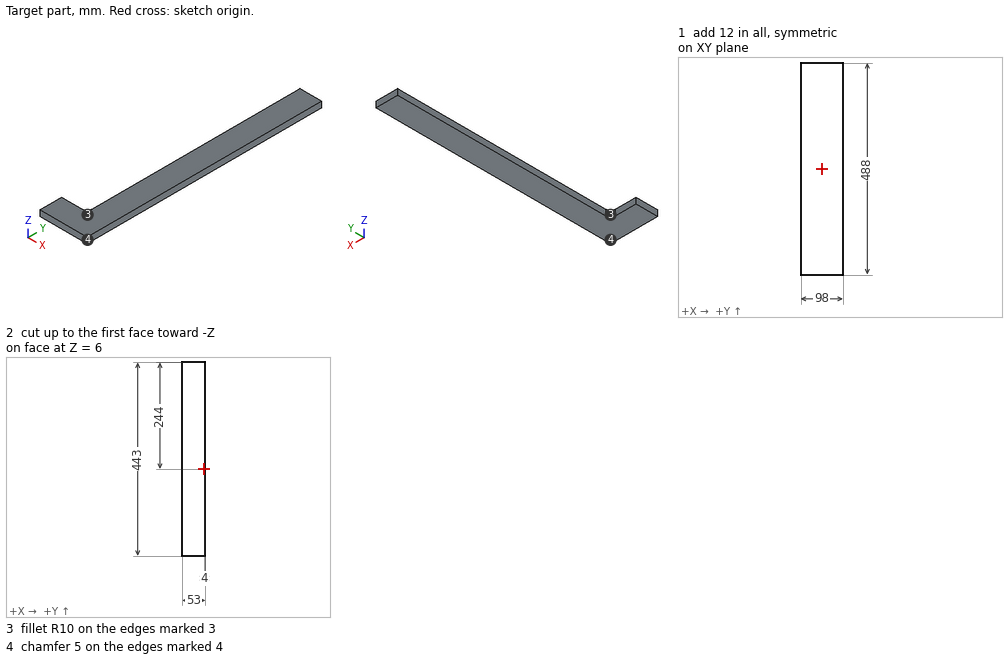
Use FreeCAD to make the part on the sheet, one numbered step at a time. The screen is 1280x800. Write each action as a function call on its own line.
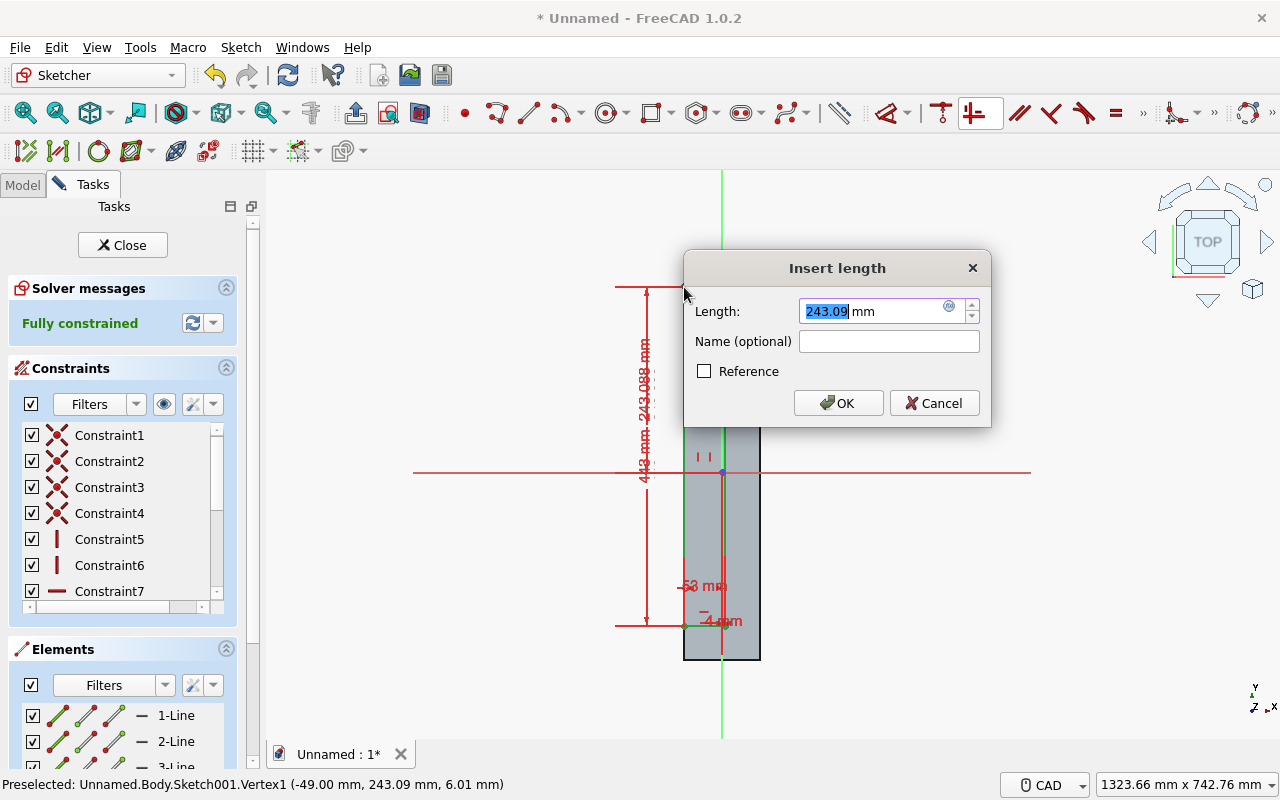
text(244)
key(Return)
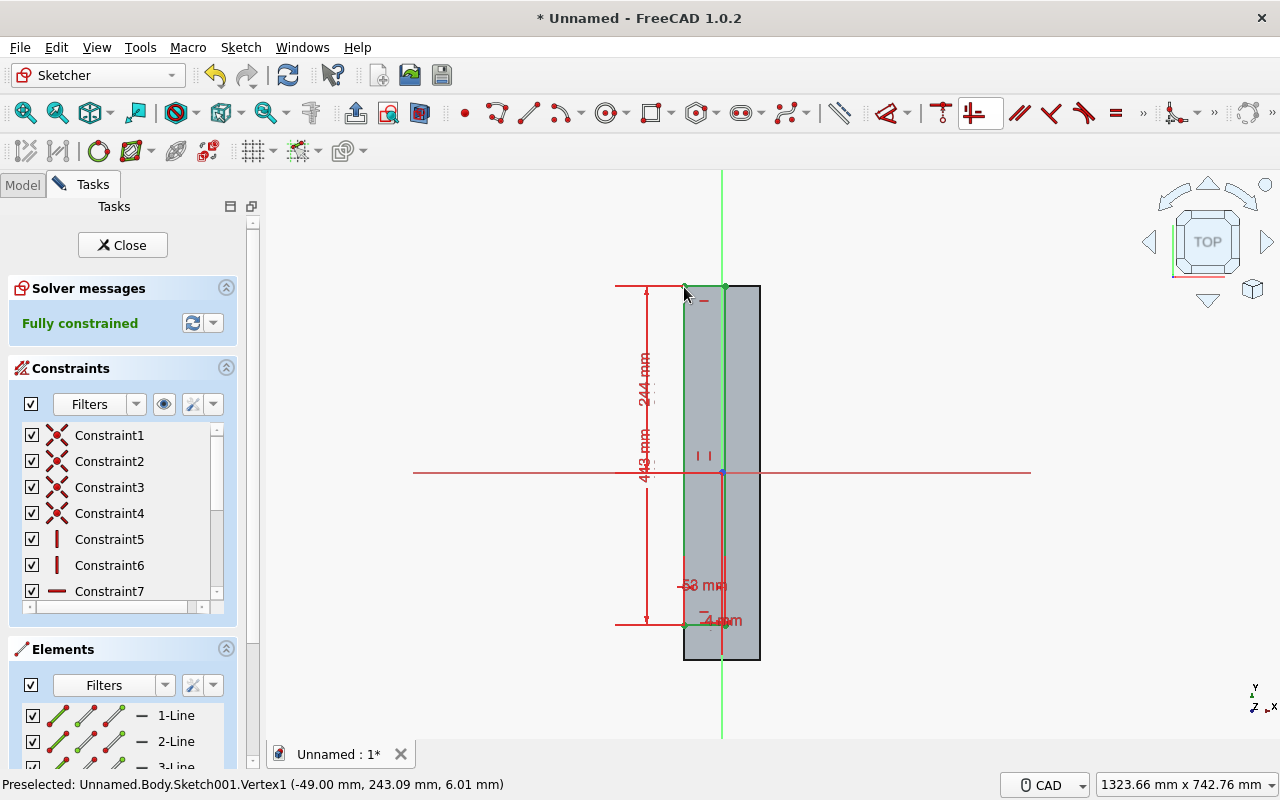
click(123, 245)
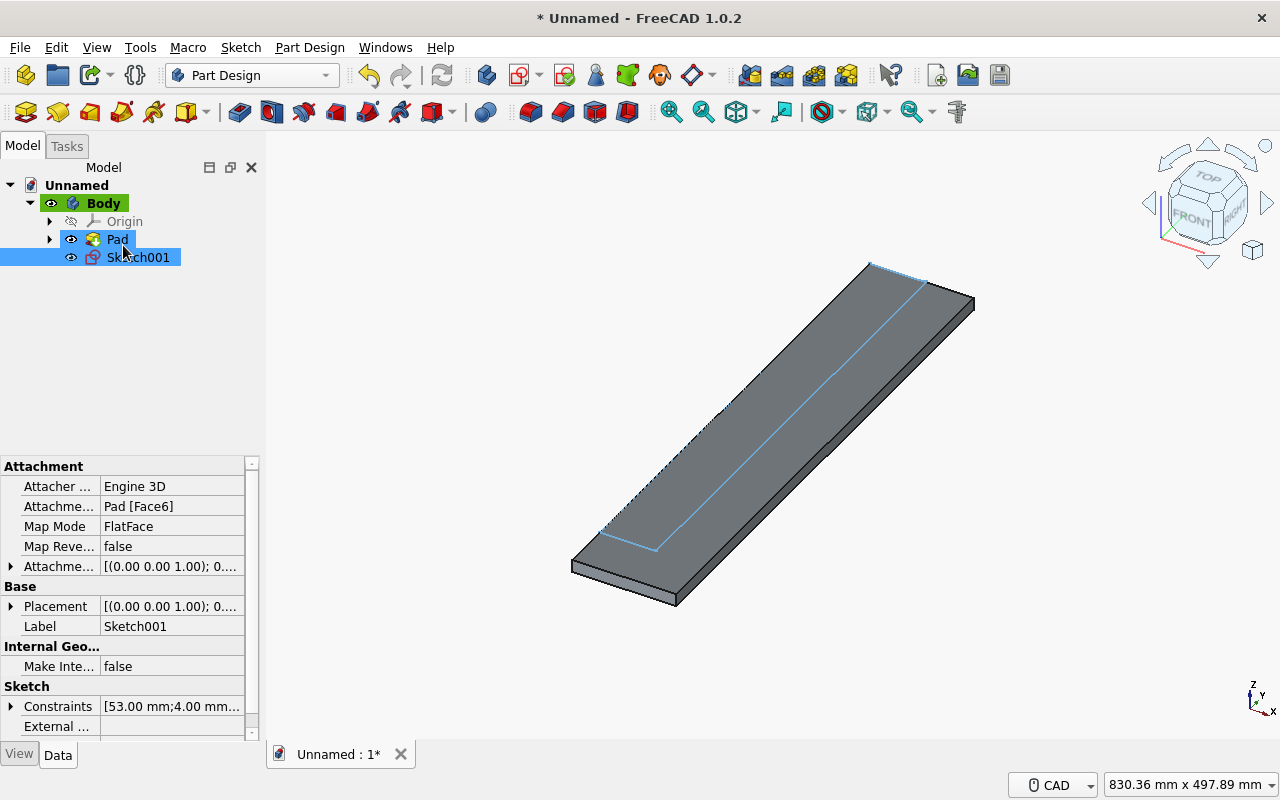
click(240, 112)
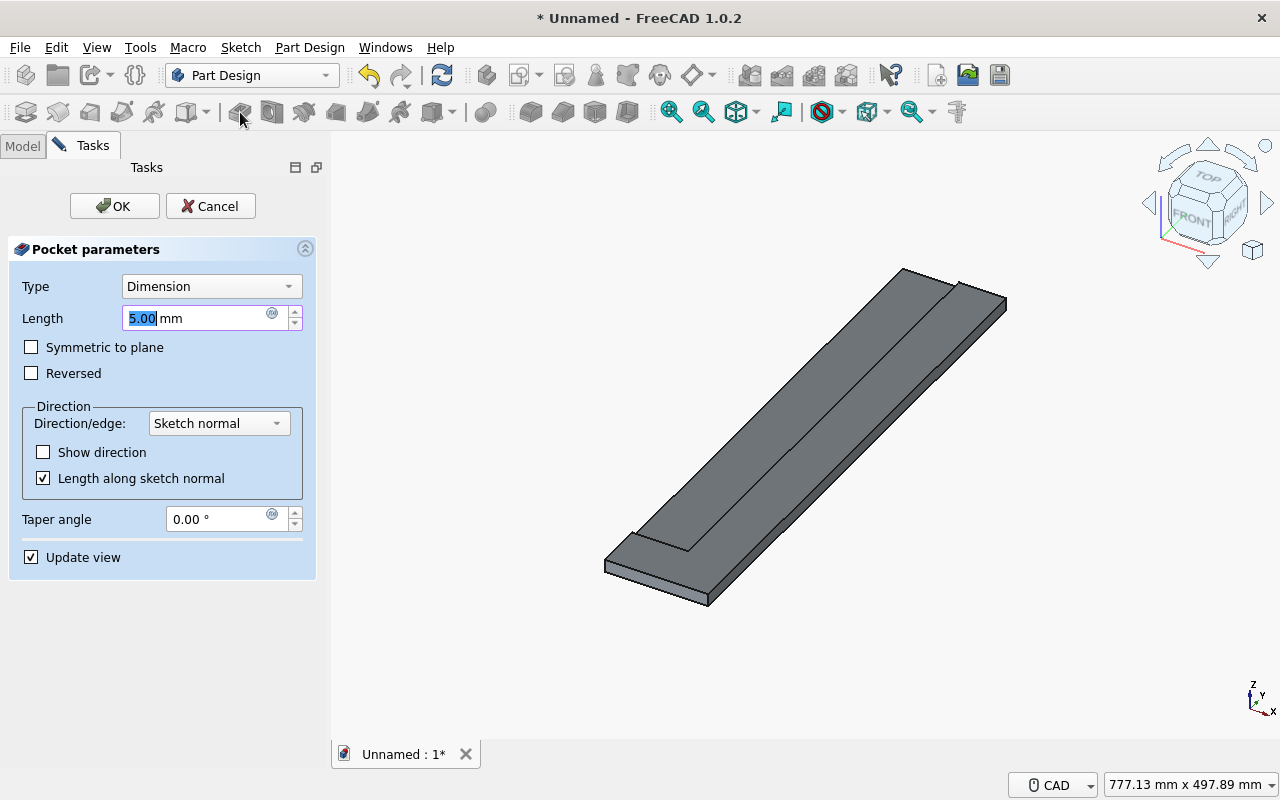
click(212, 286)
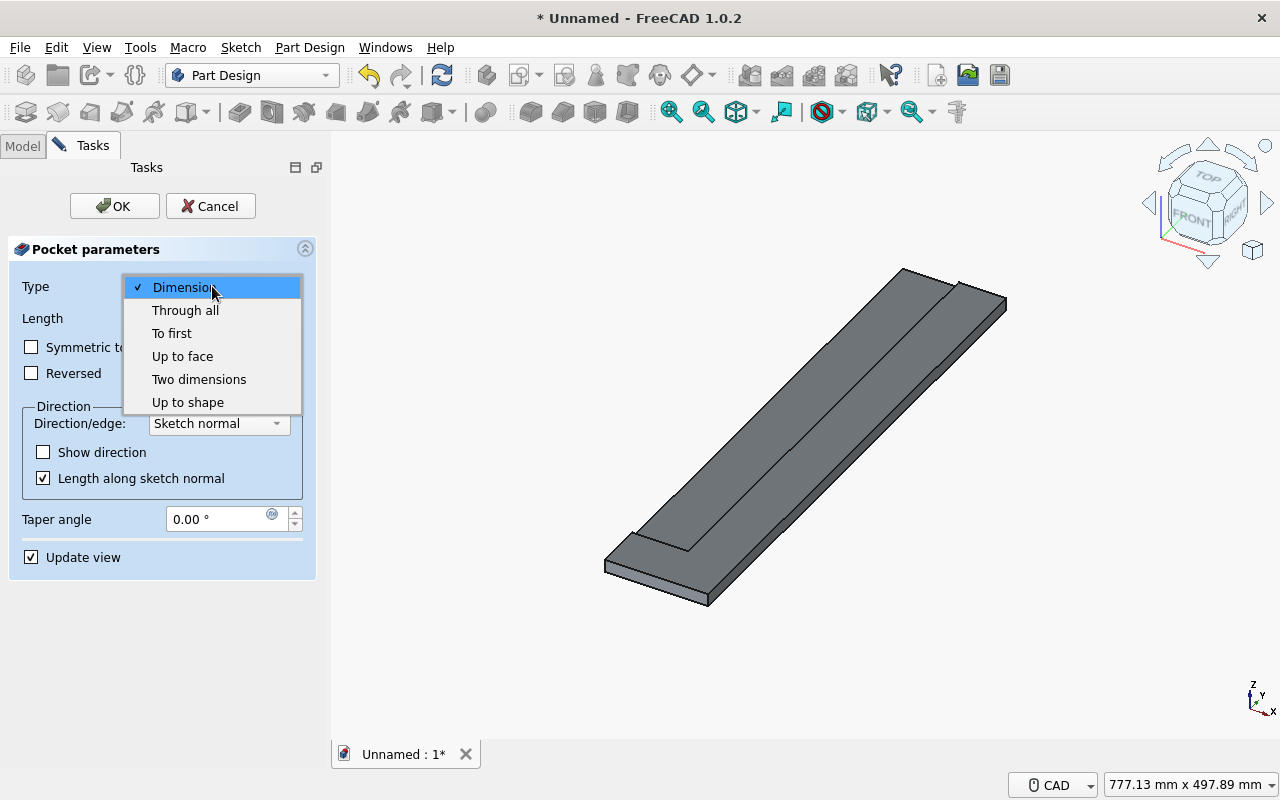
click(212, 334)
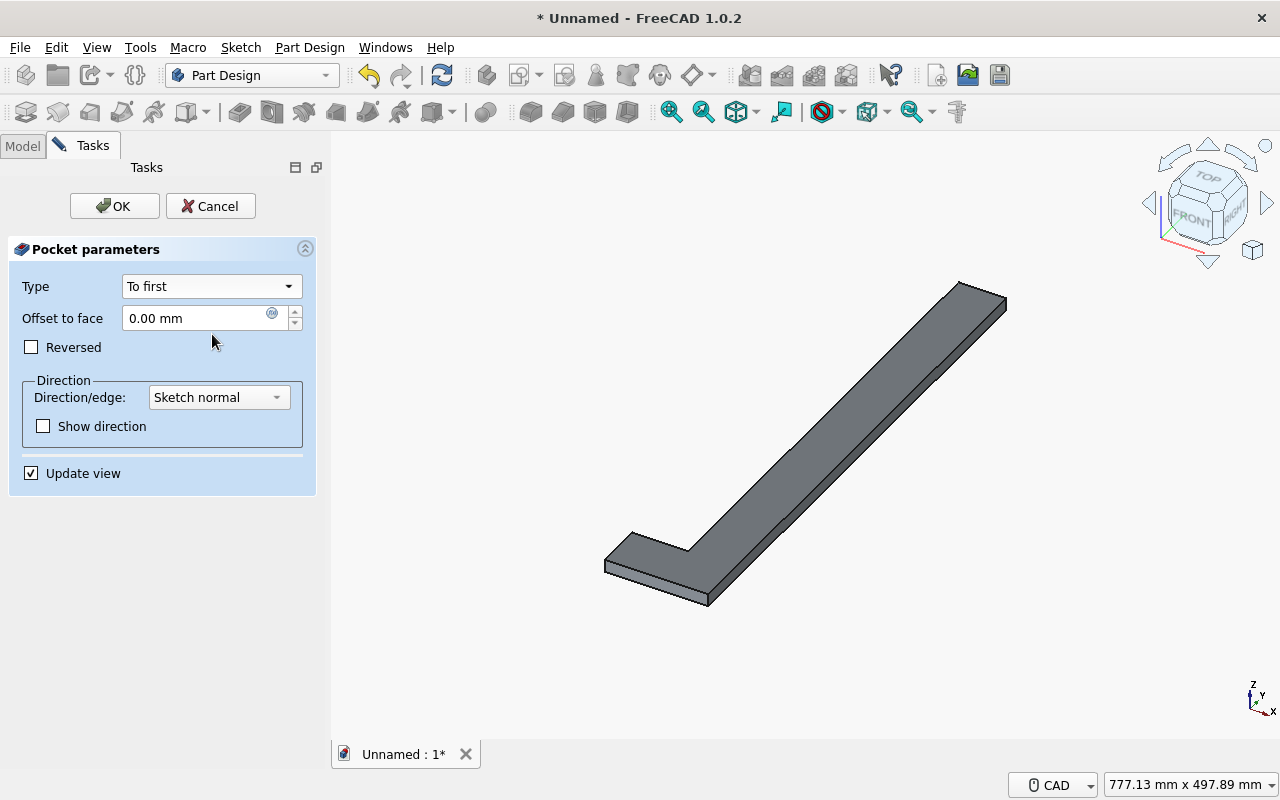
click(115, 206)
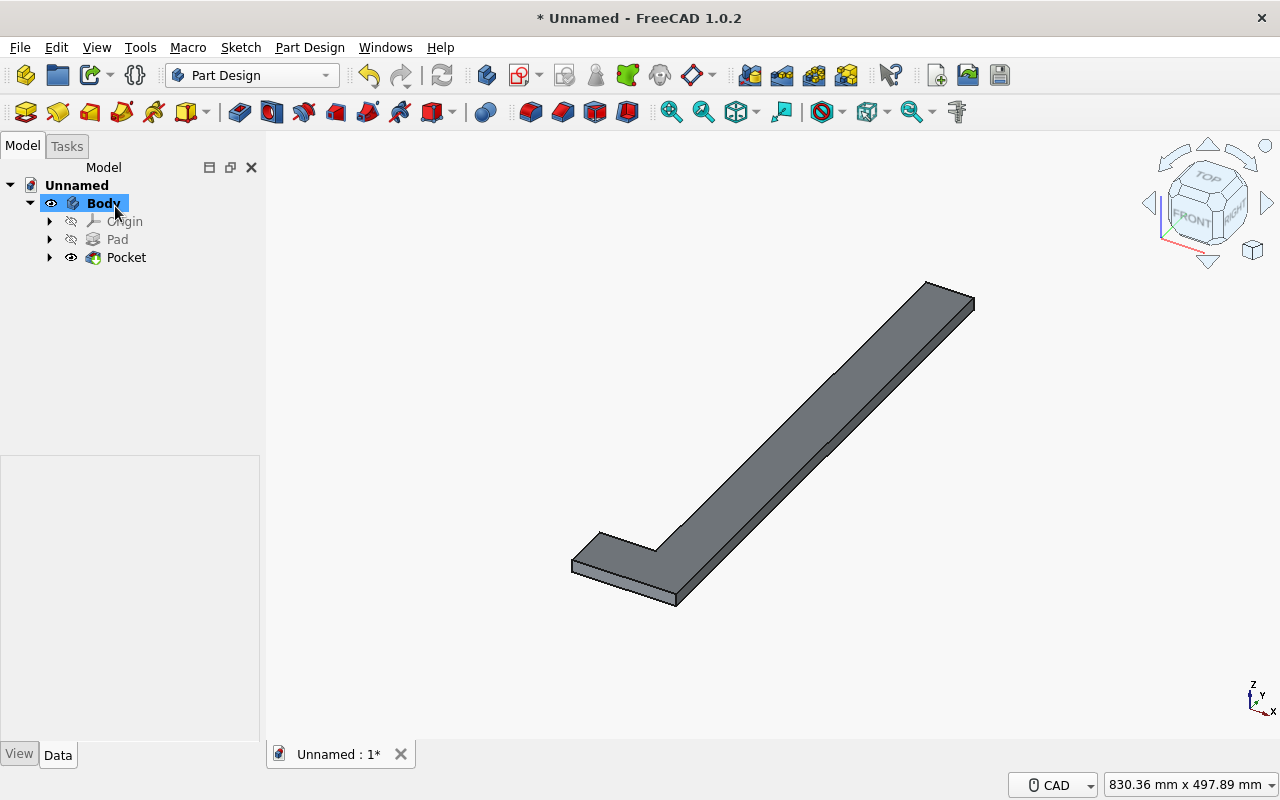
scroll(656, 556, up, 6)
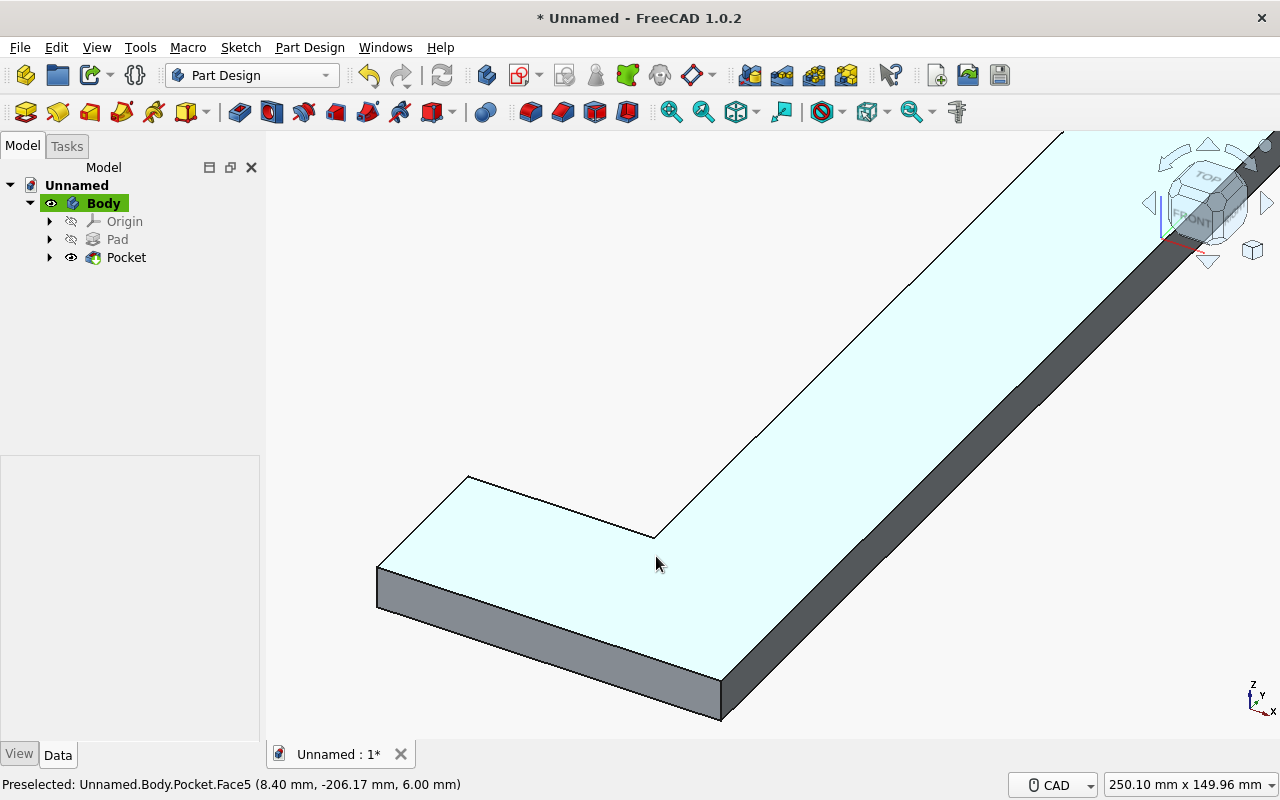
key(v)
key(f)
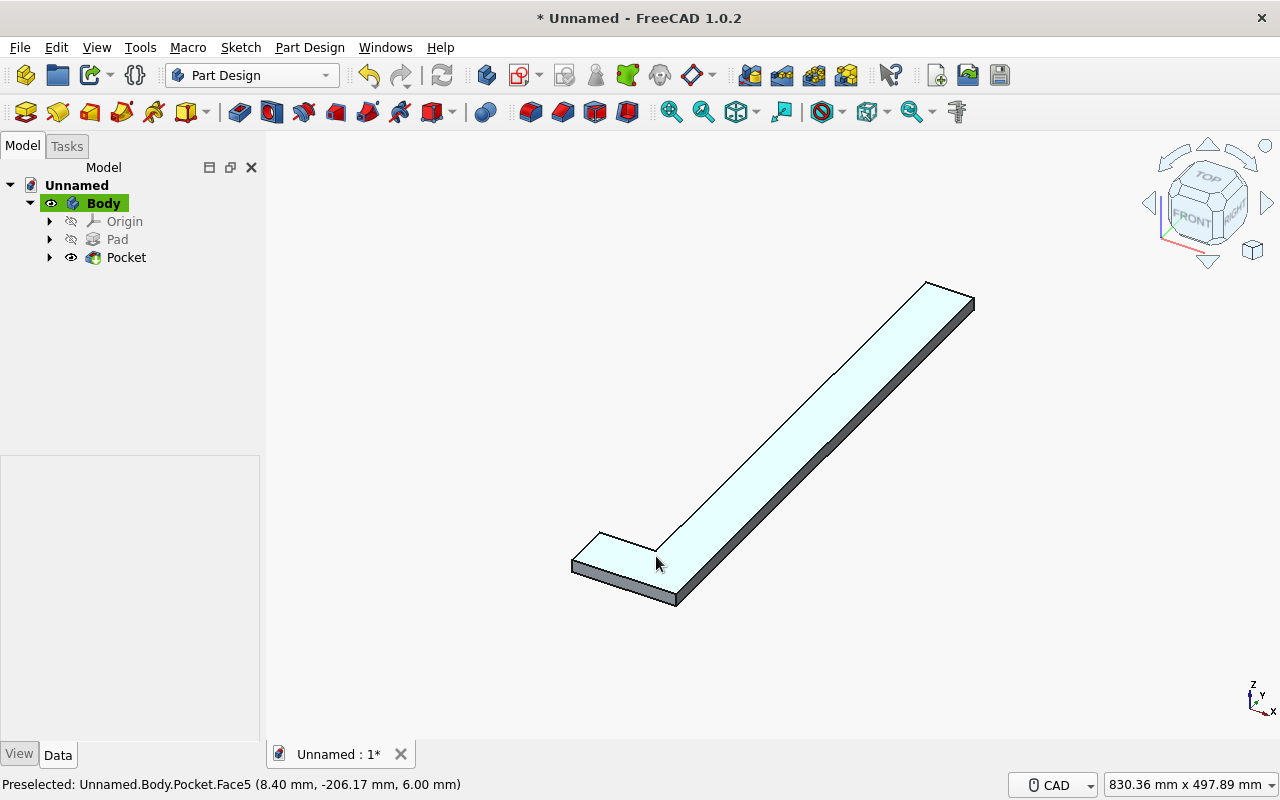
key(0)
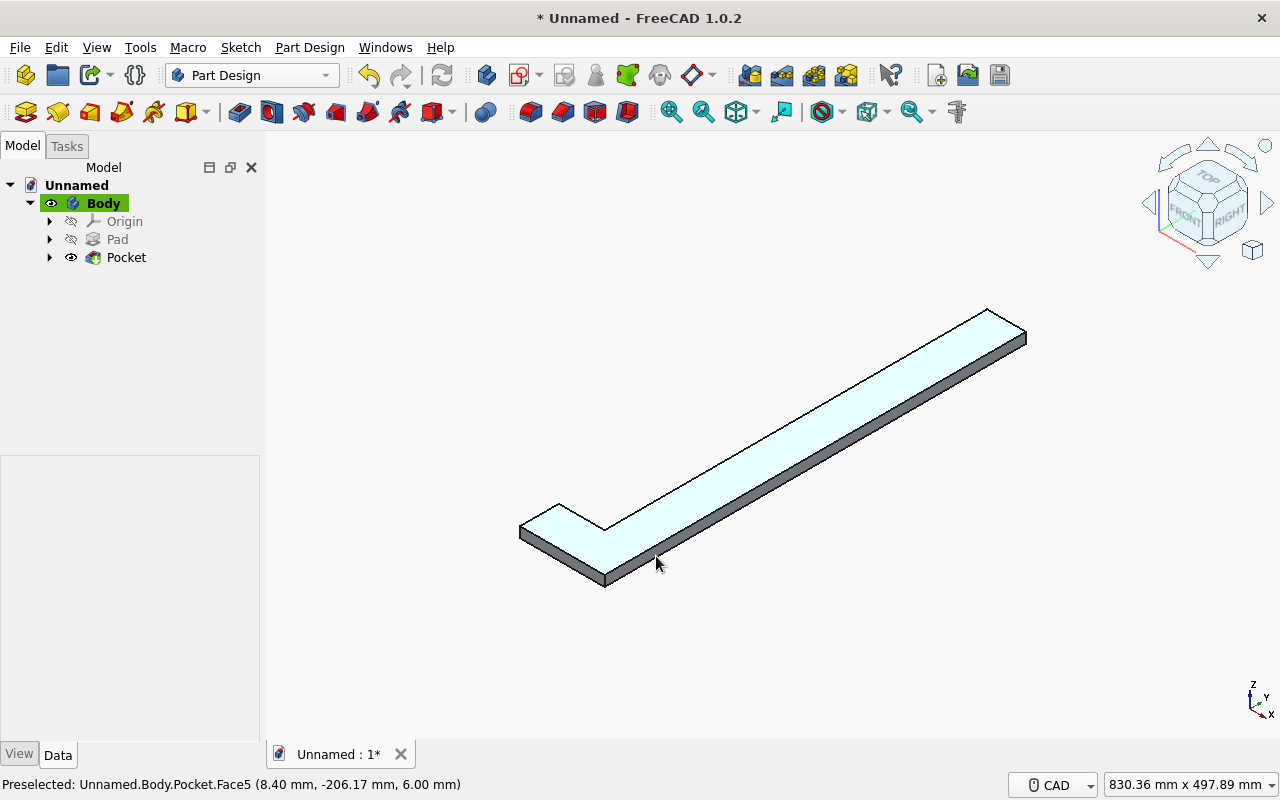
scroll(605, 535, up, 6)